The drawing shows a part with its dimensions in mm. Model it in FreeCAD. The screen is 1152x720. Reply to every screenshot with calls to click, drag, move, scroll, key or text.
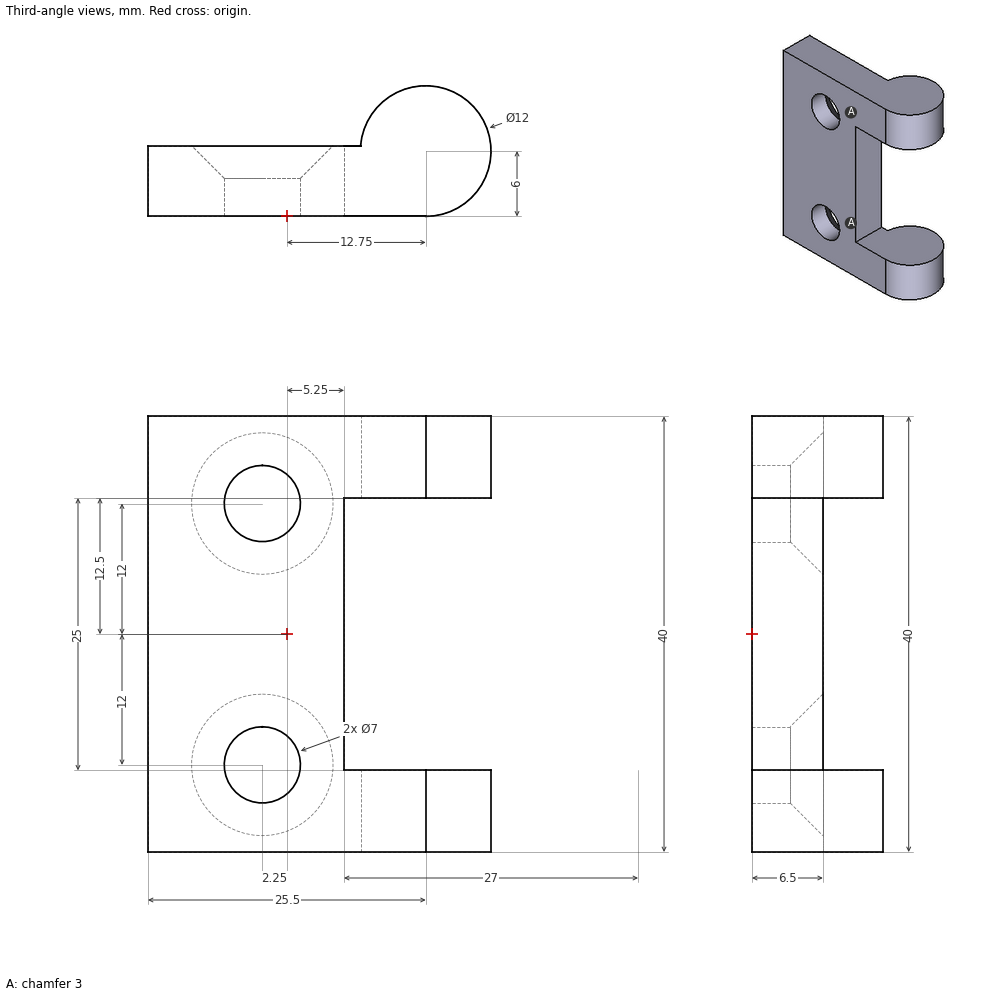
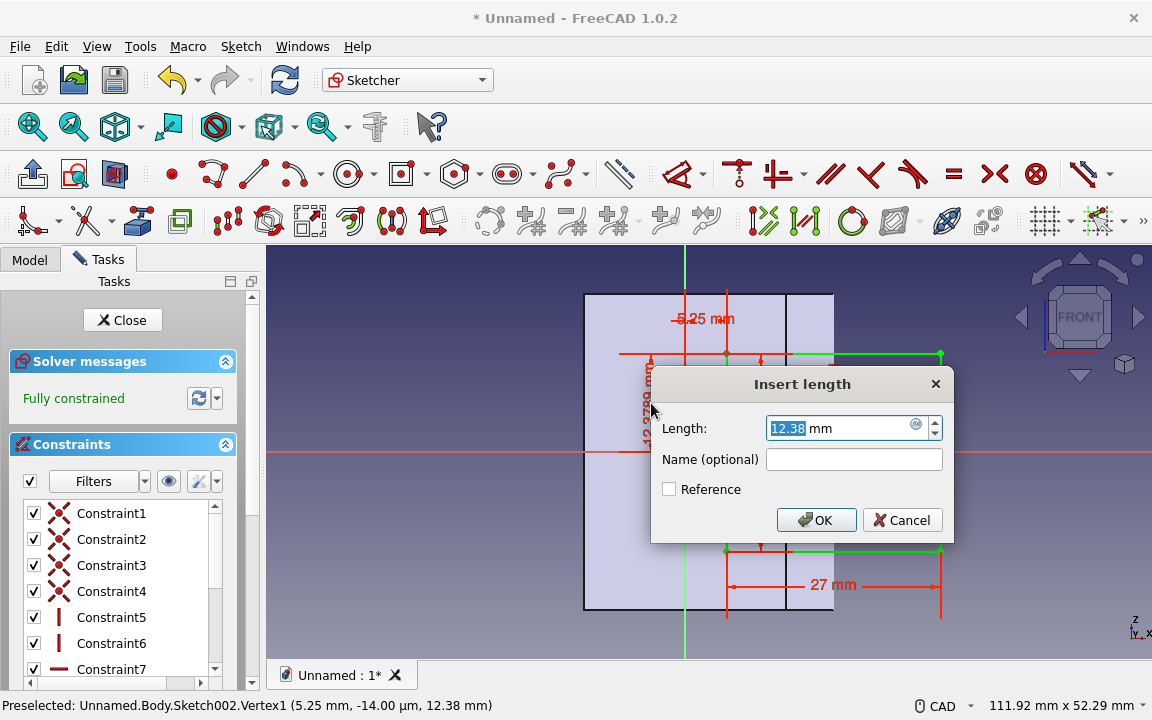
text(12.5)
key(Return)
key(Escape)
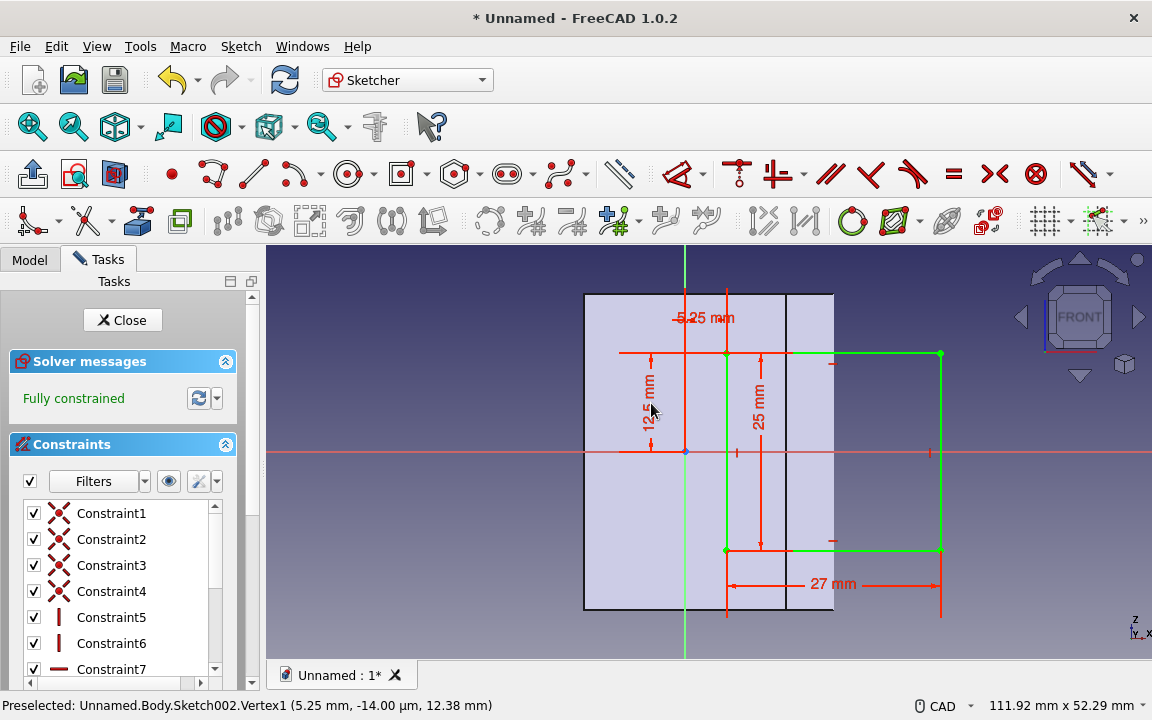
click(123, 320)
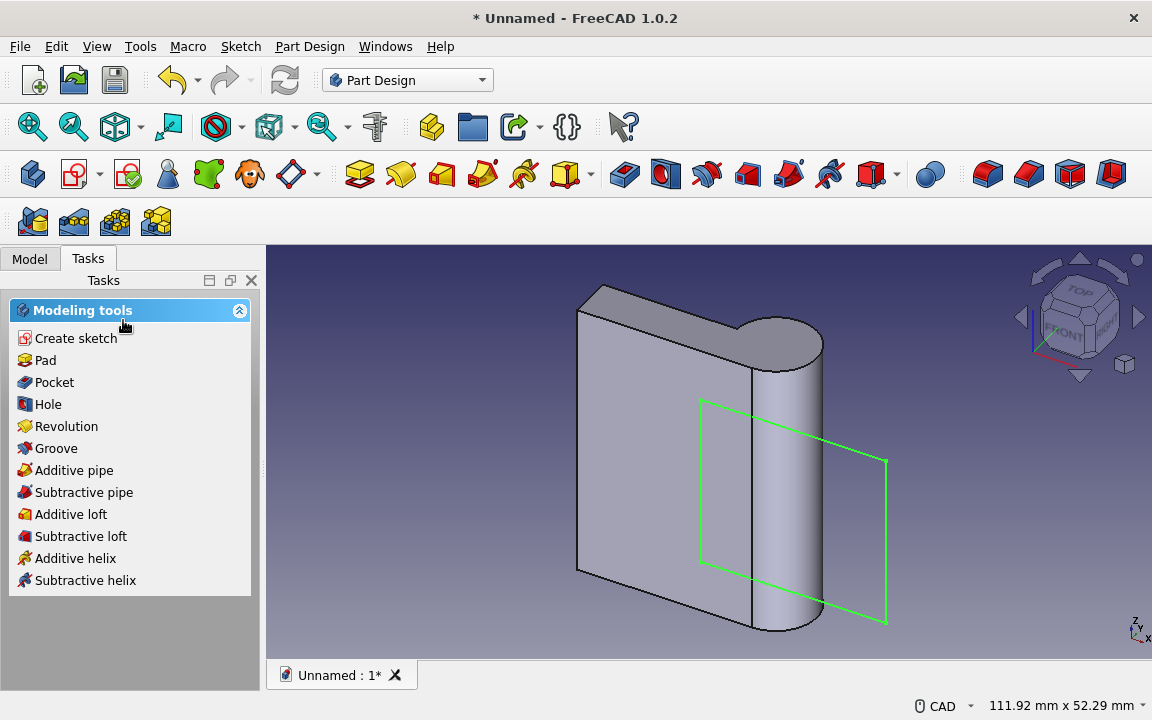
click(625, 174)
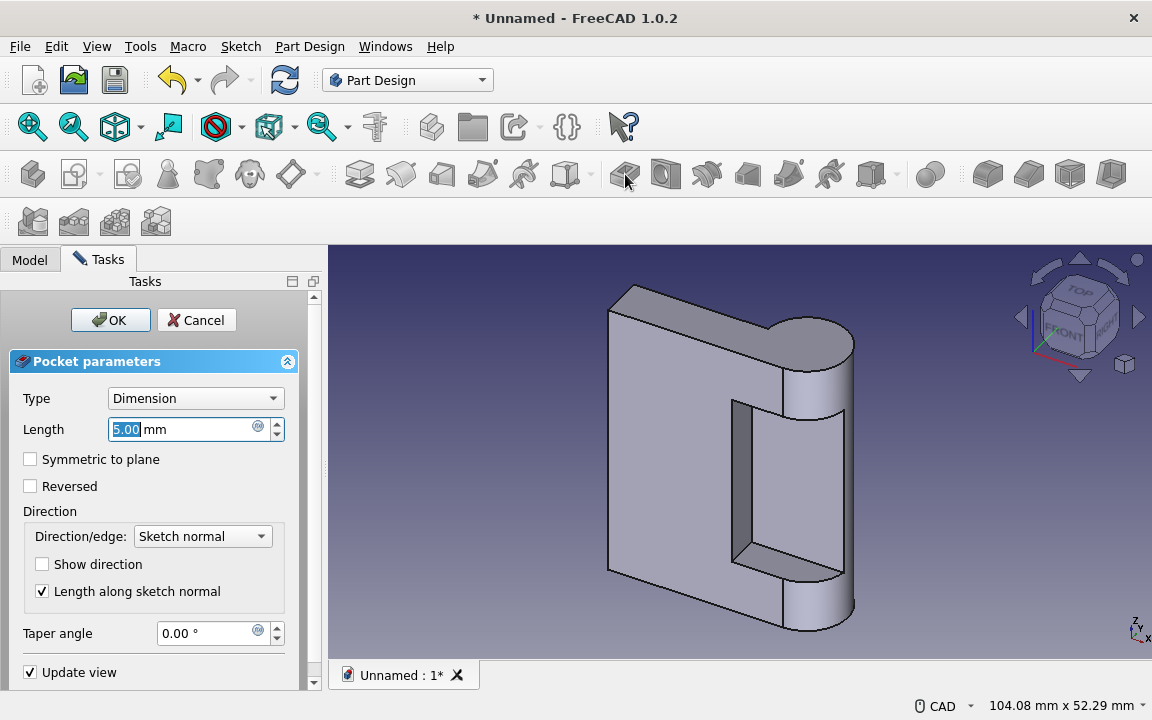
click(196, 398)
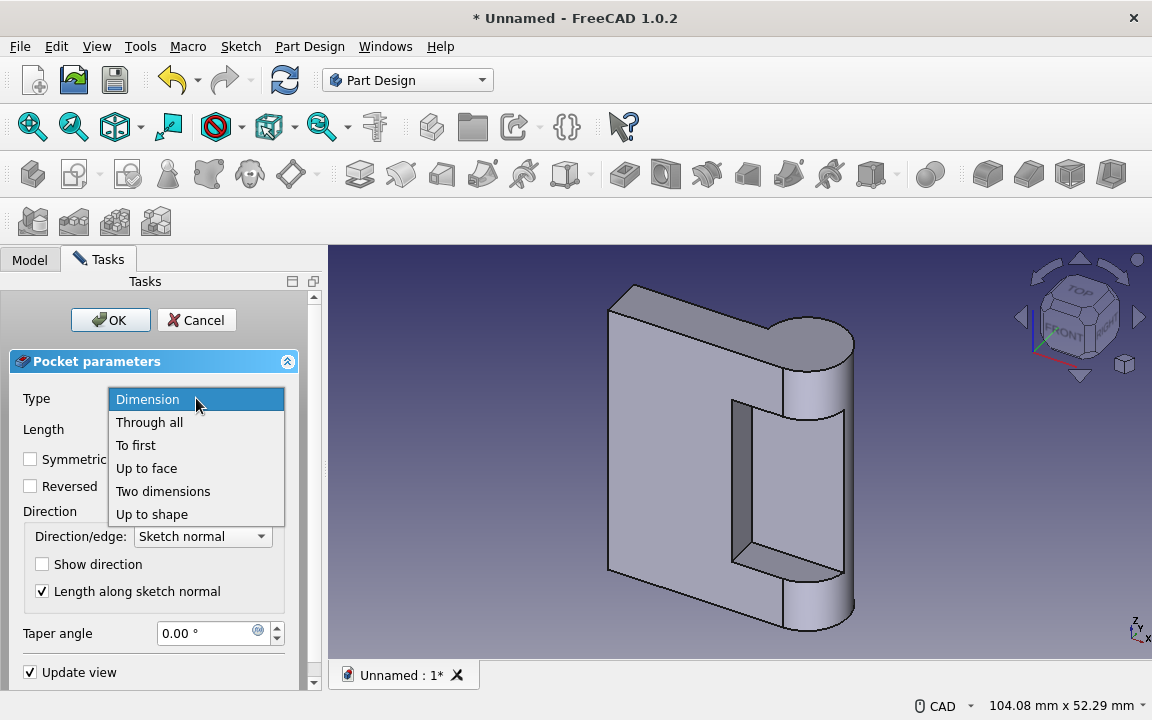
click(194, 422)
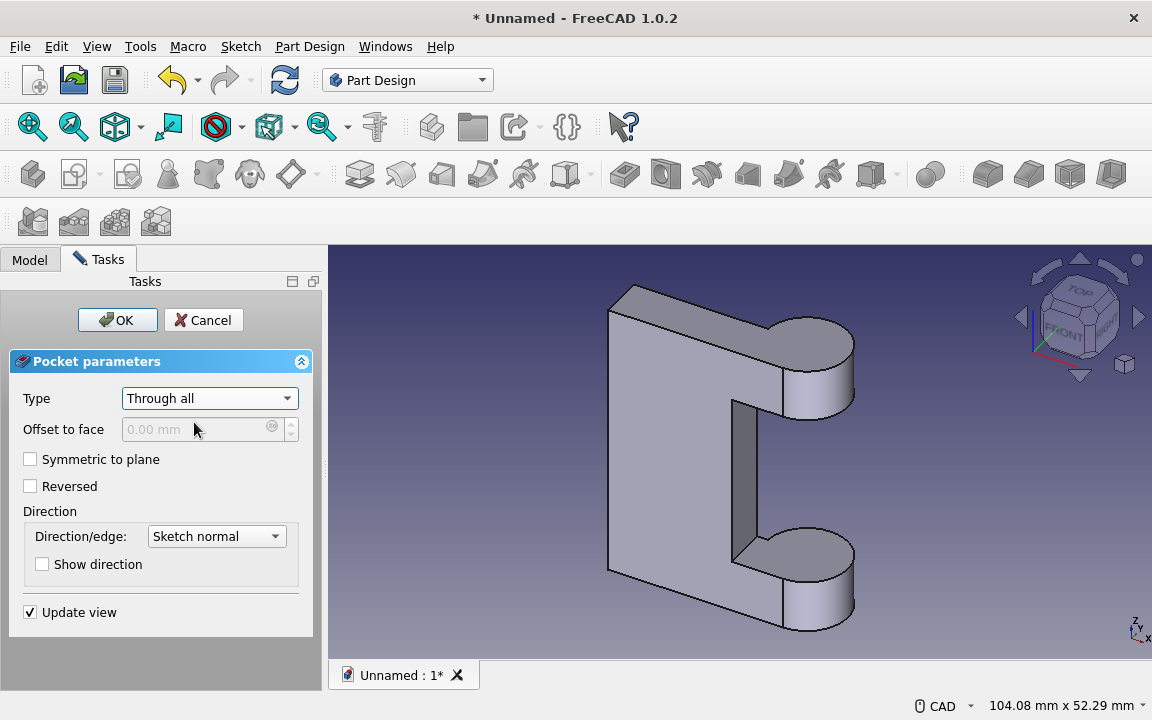
click(118, 320)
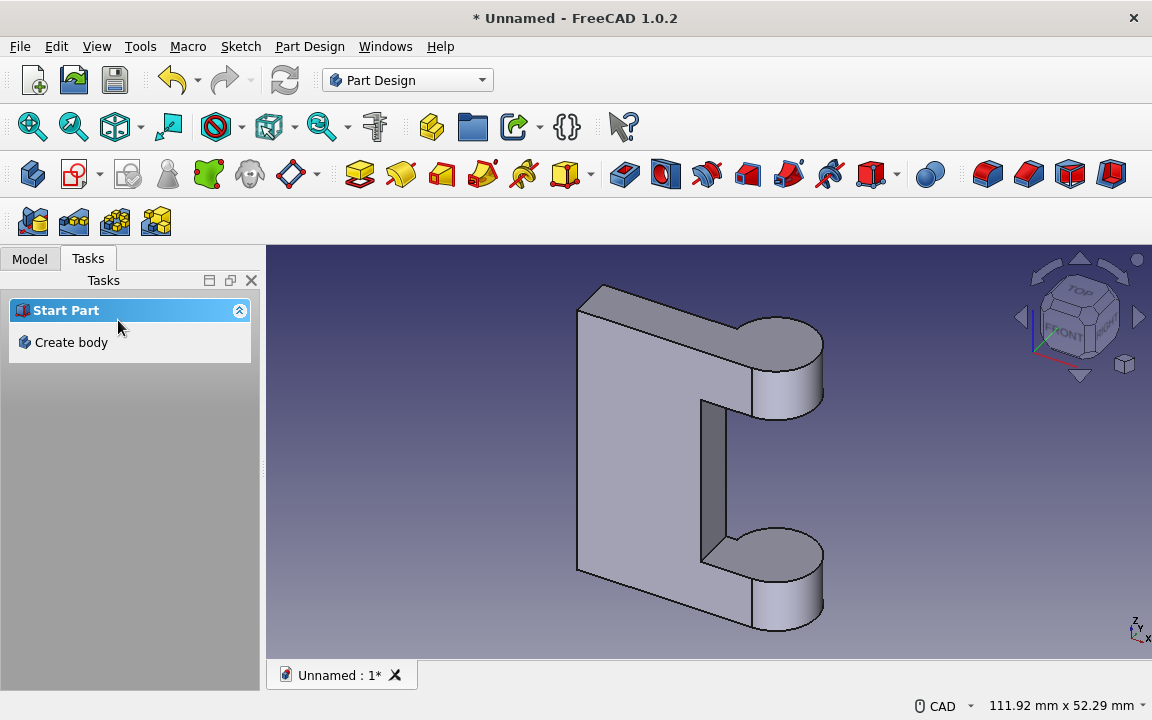
key(4)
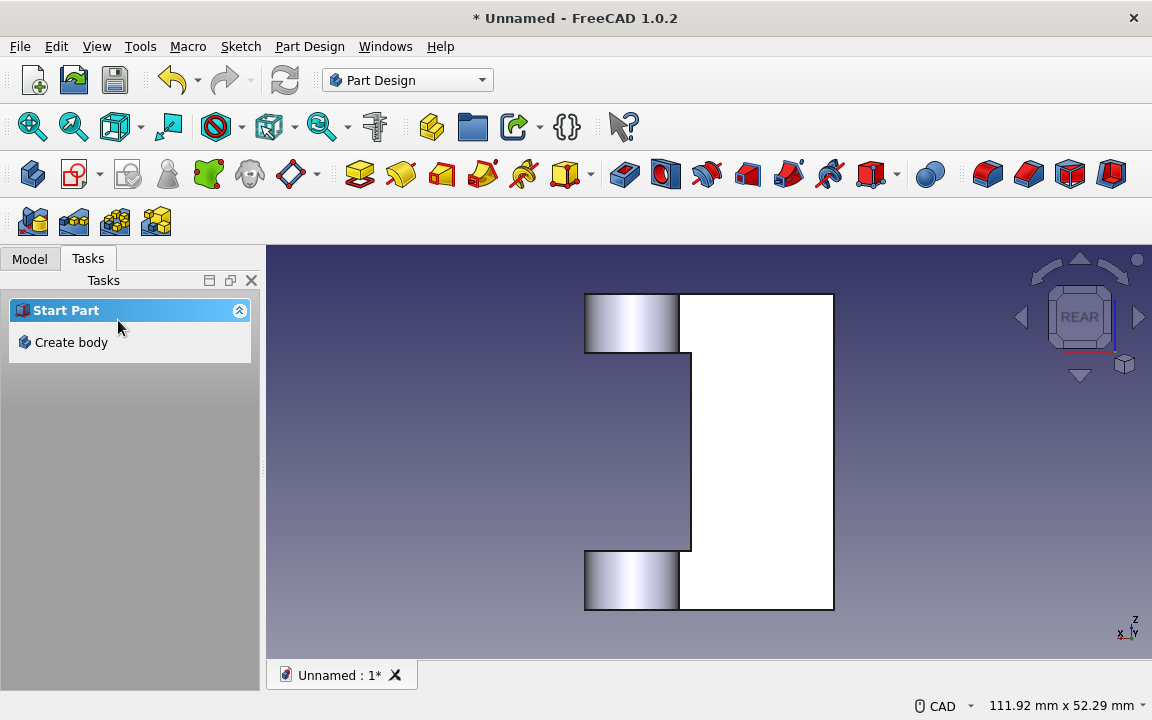
click(756, 361)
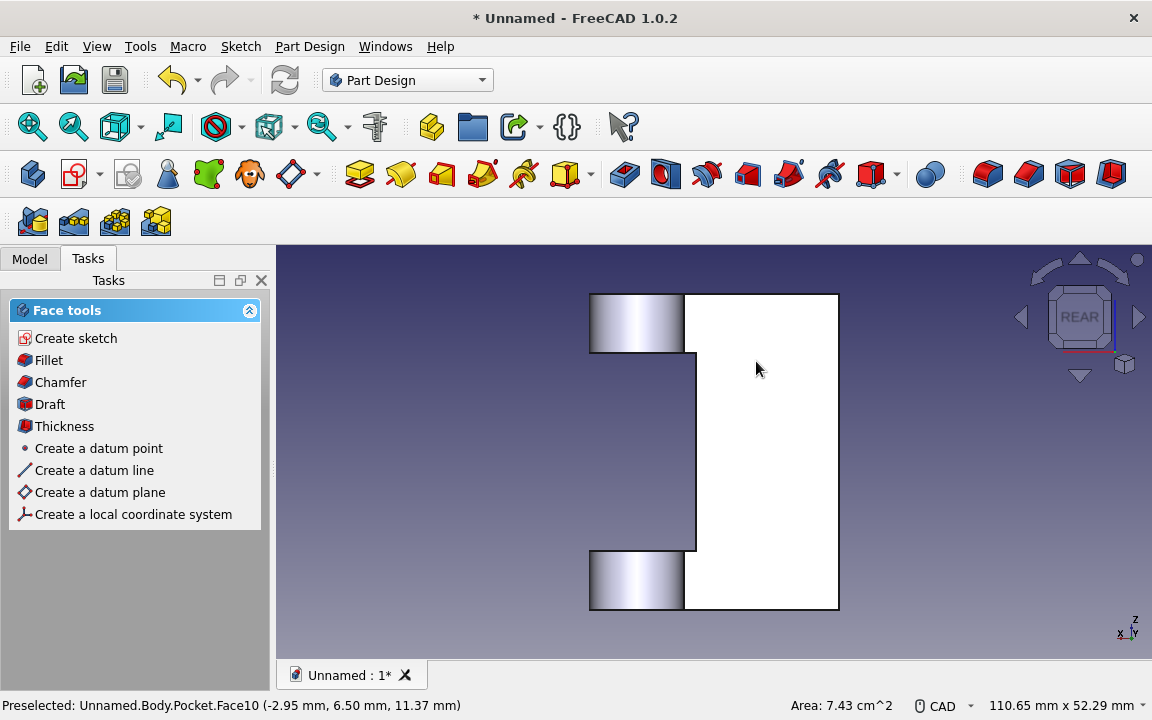
click(74, 174)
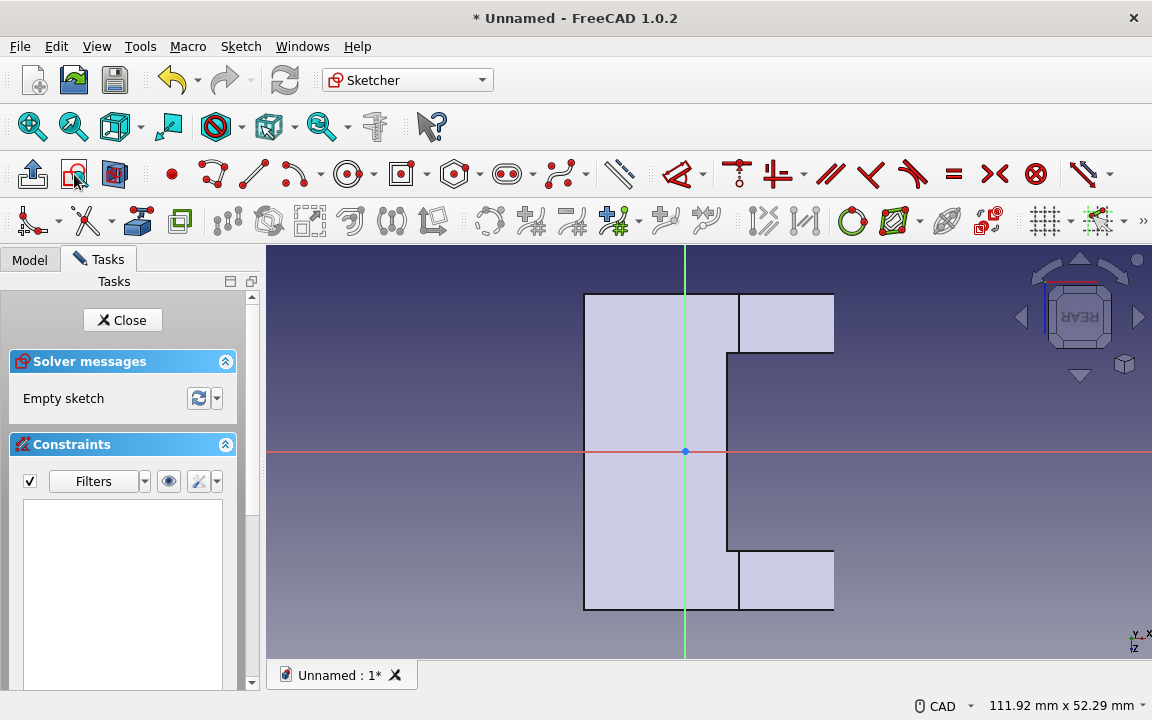
click(115, 174)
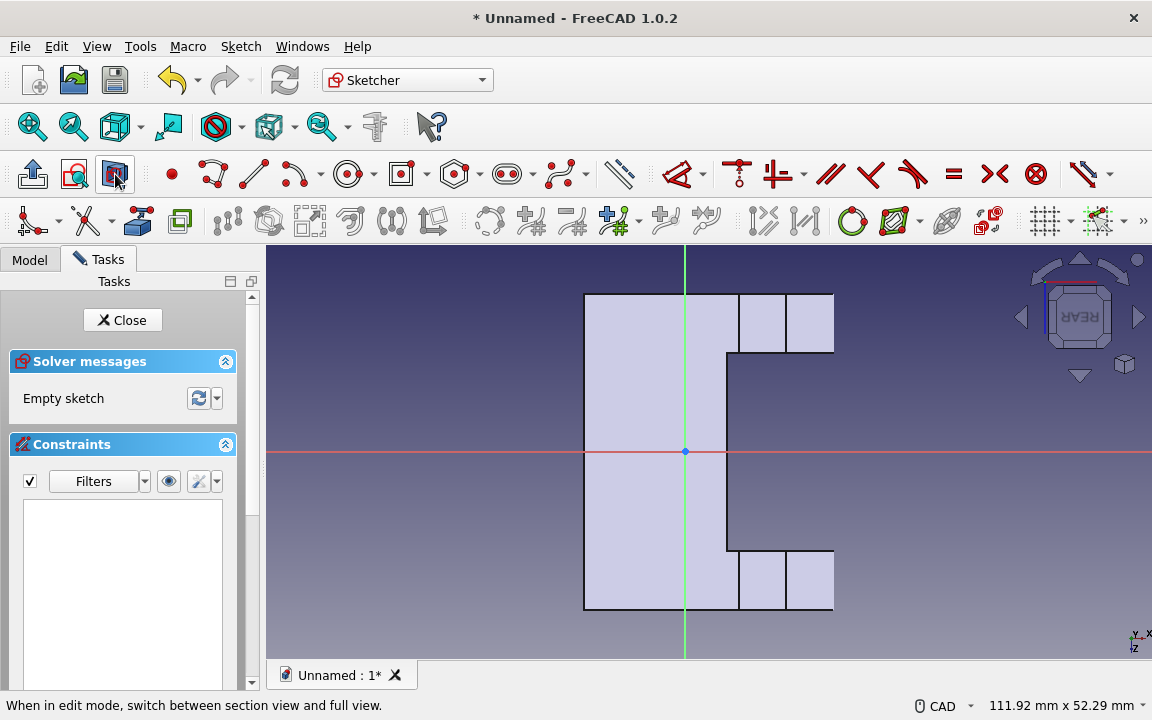
click(348, 174)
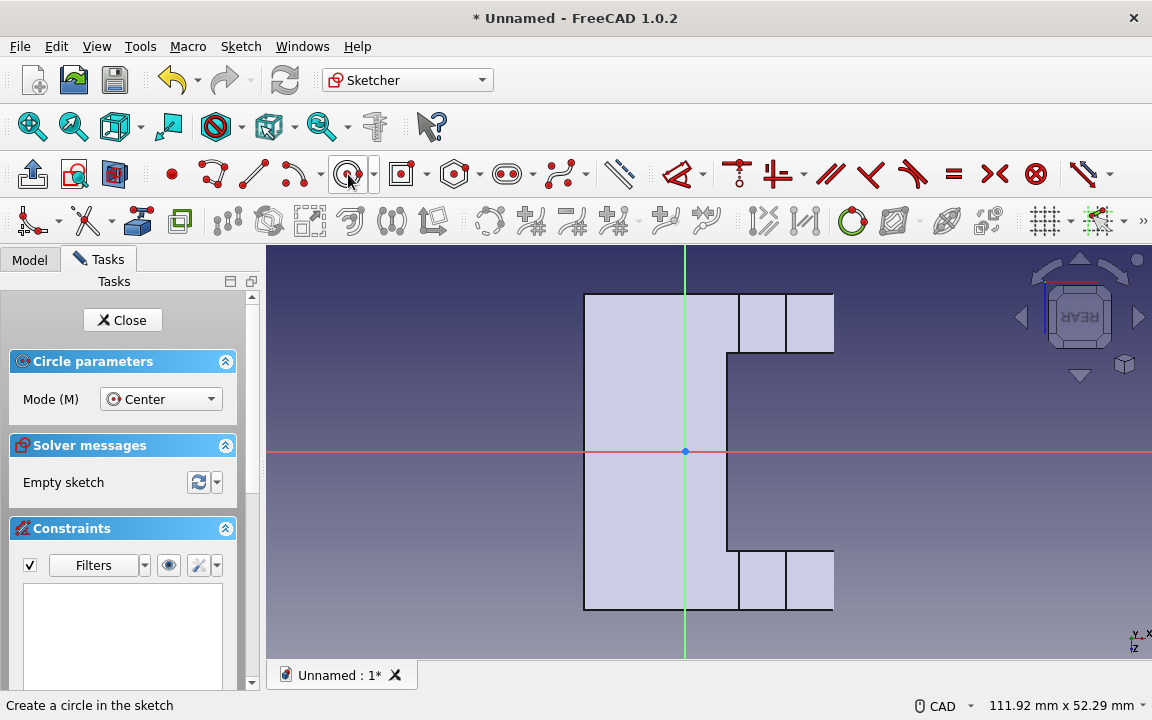
click(668, 357)
click(648, 337)